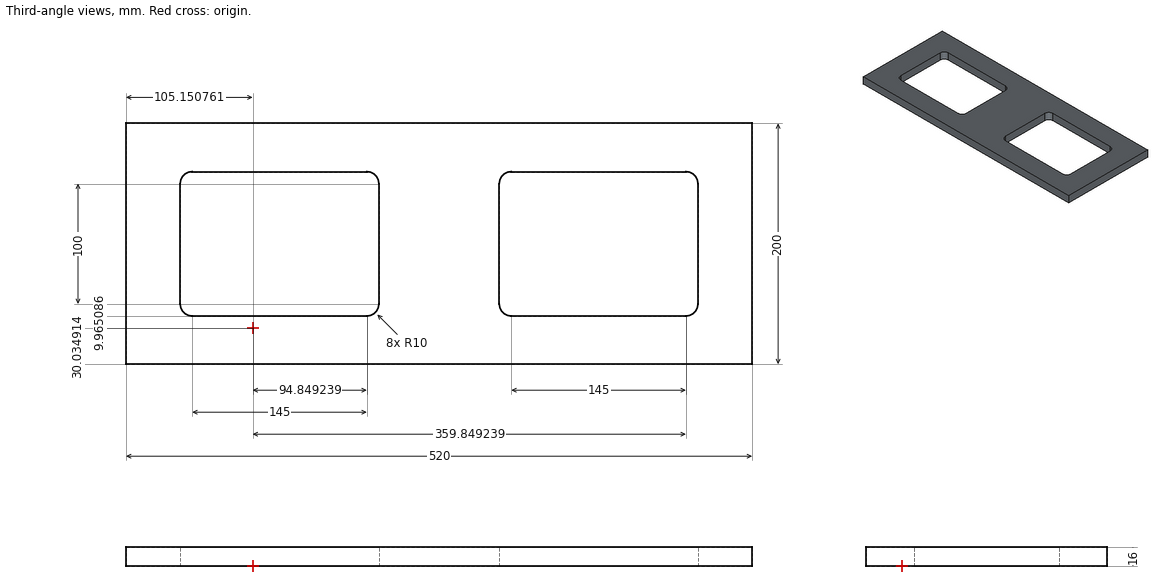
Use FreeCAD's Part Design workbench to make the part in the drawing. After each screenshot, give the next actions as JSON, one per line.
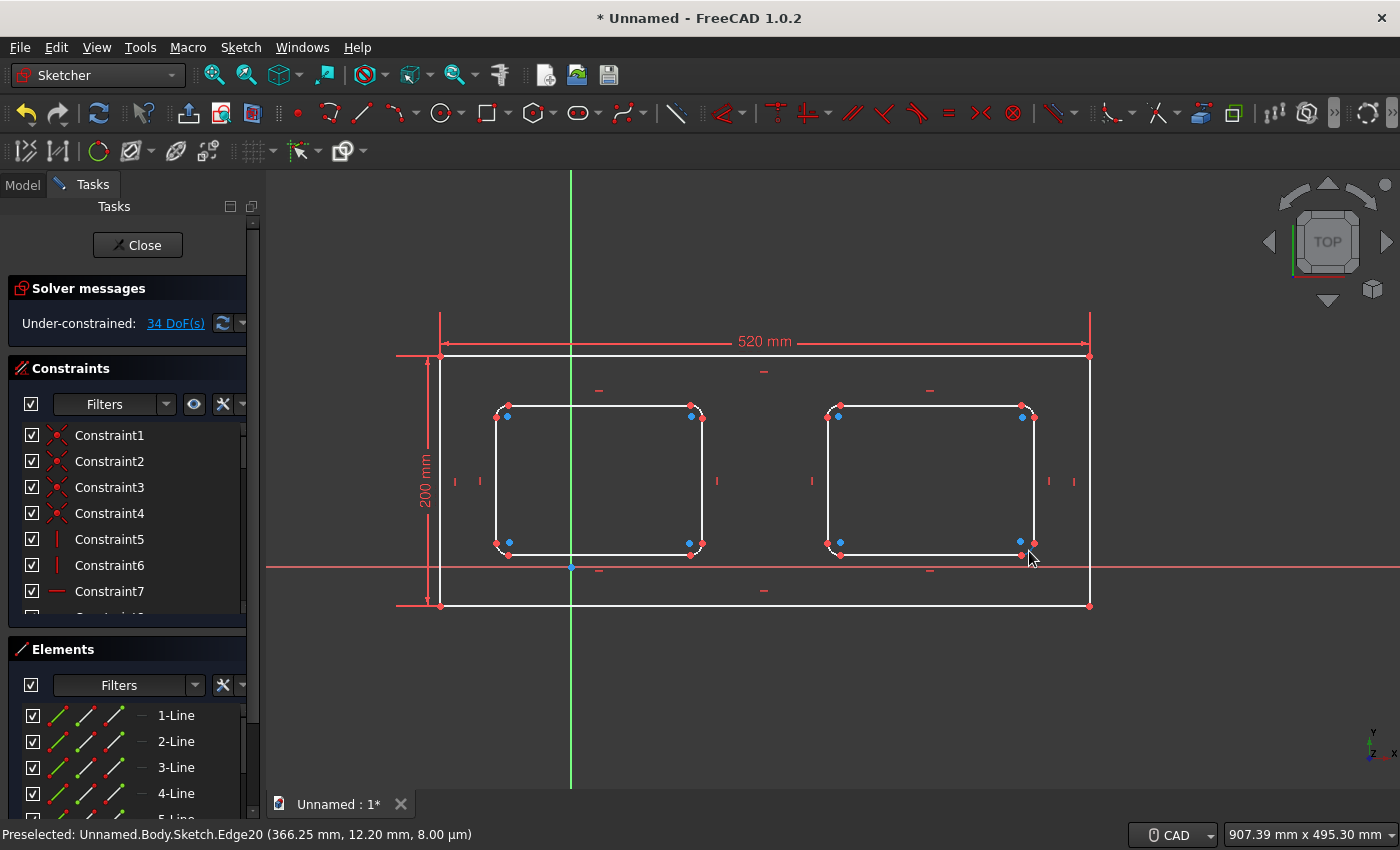
{"action": "left_click", "coordinate": [702, 456]}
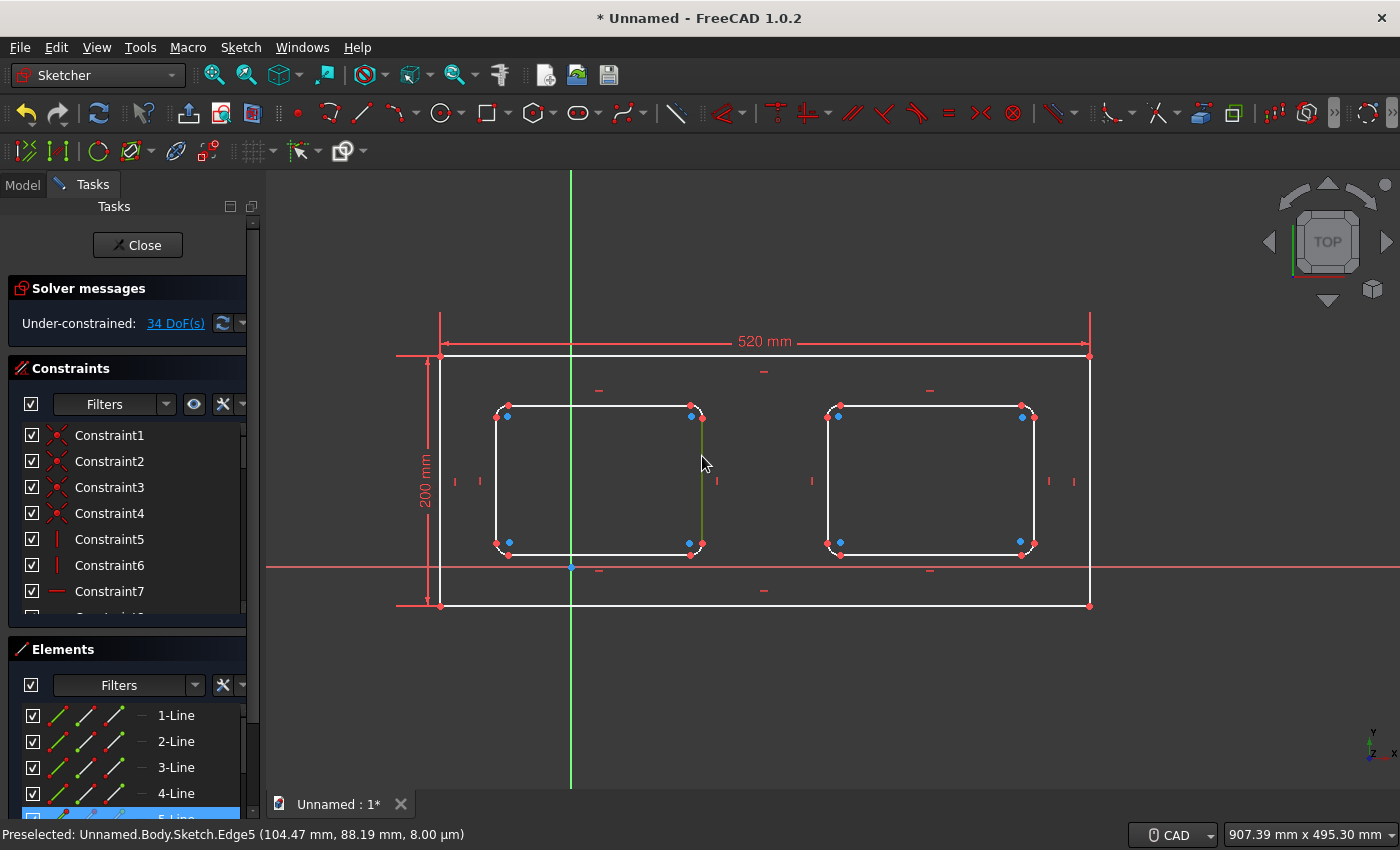
{"action": "scroll", "coordinate": [699, 552], "scroll_direction": "up", "scroll_amount": 3}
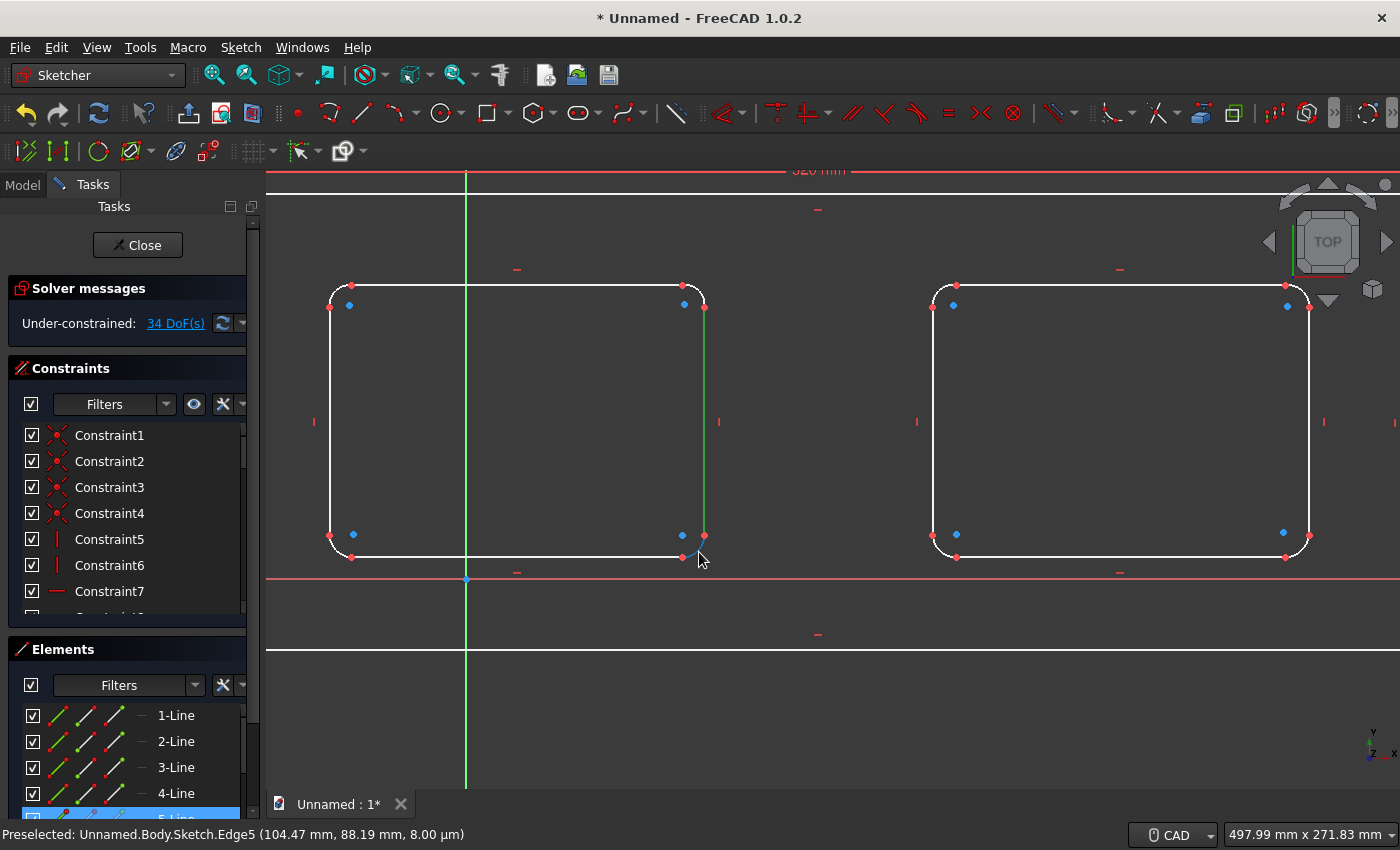
{"action": "left_click", "coordinate": [698, 551]}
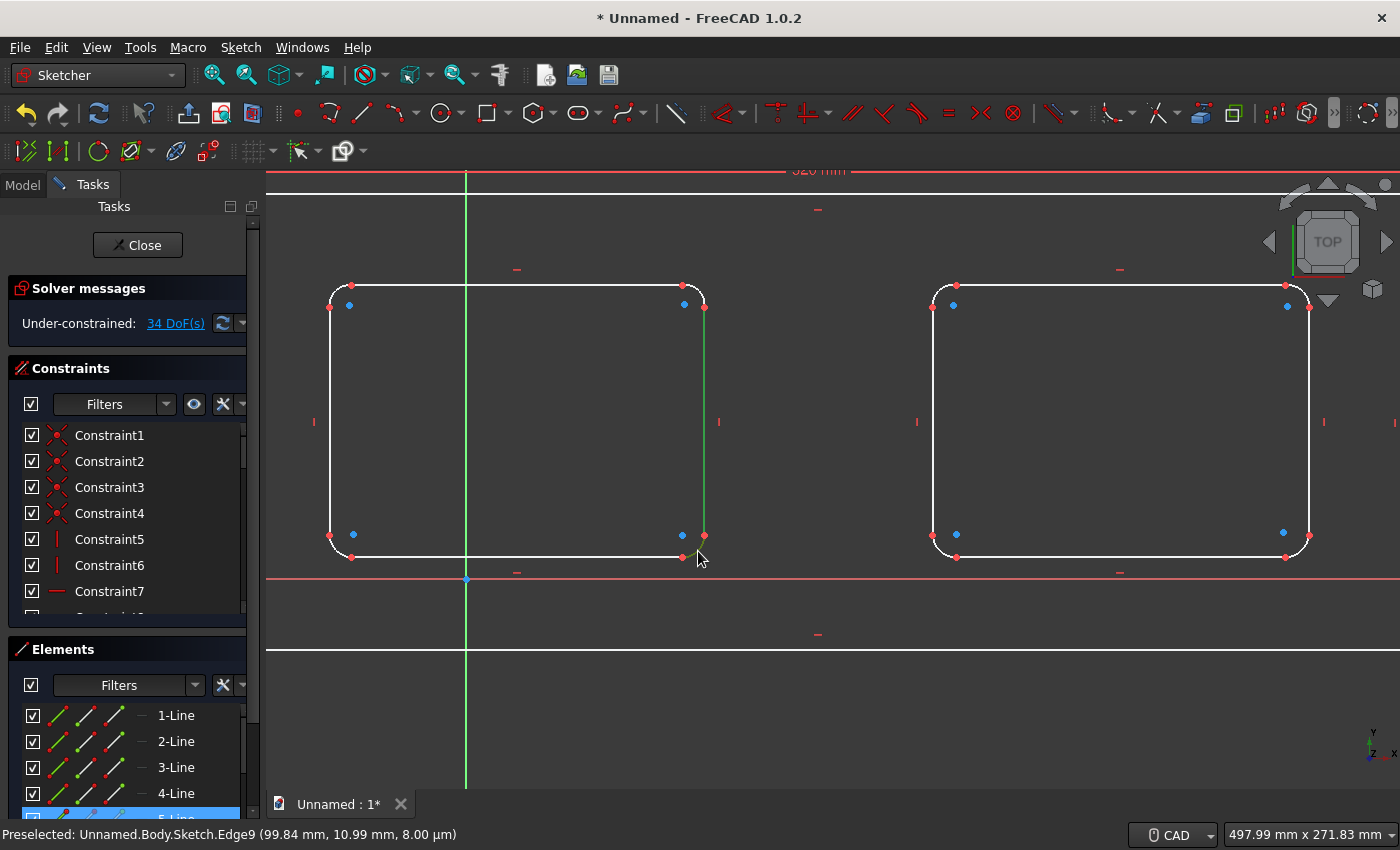
{"action": "left_click", "coordinate": [918, 114]}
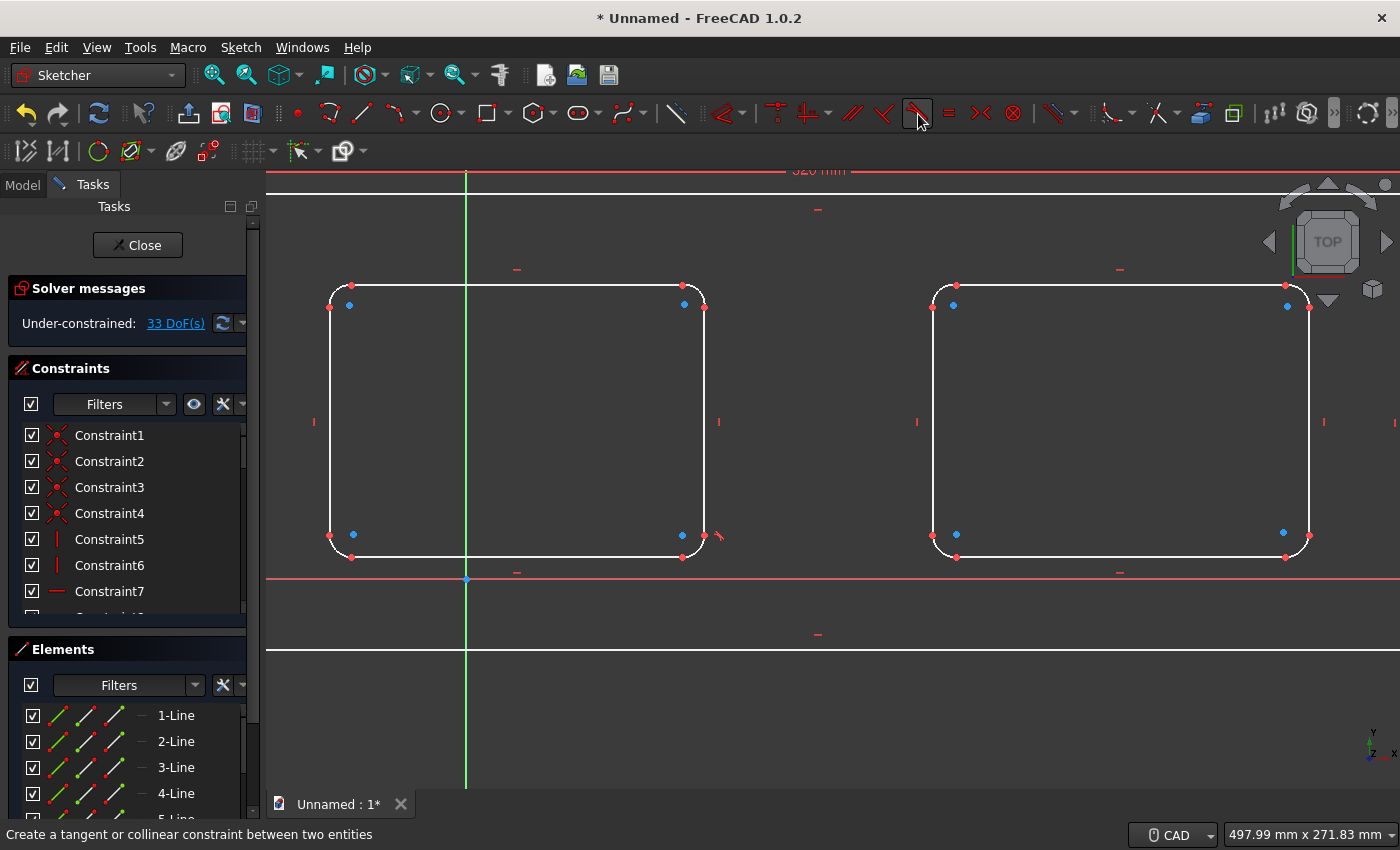
{"action": "left_click", "coordinate": [704, 376]}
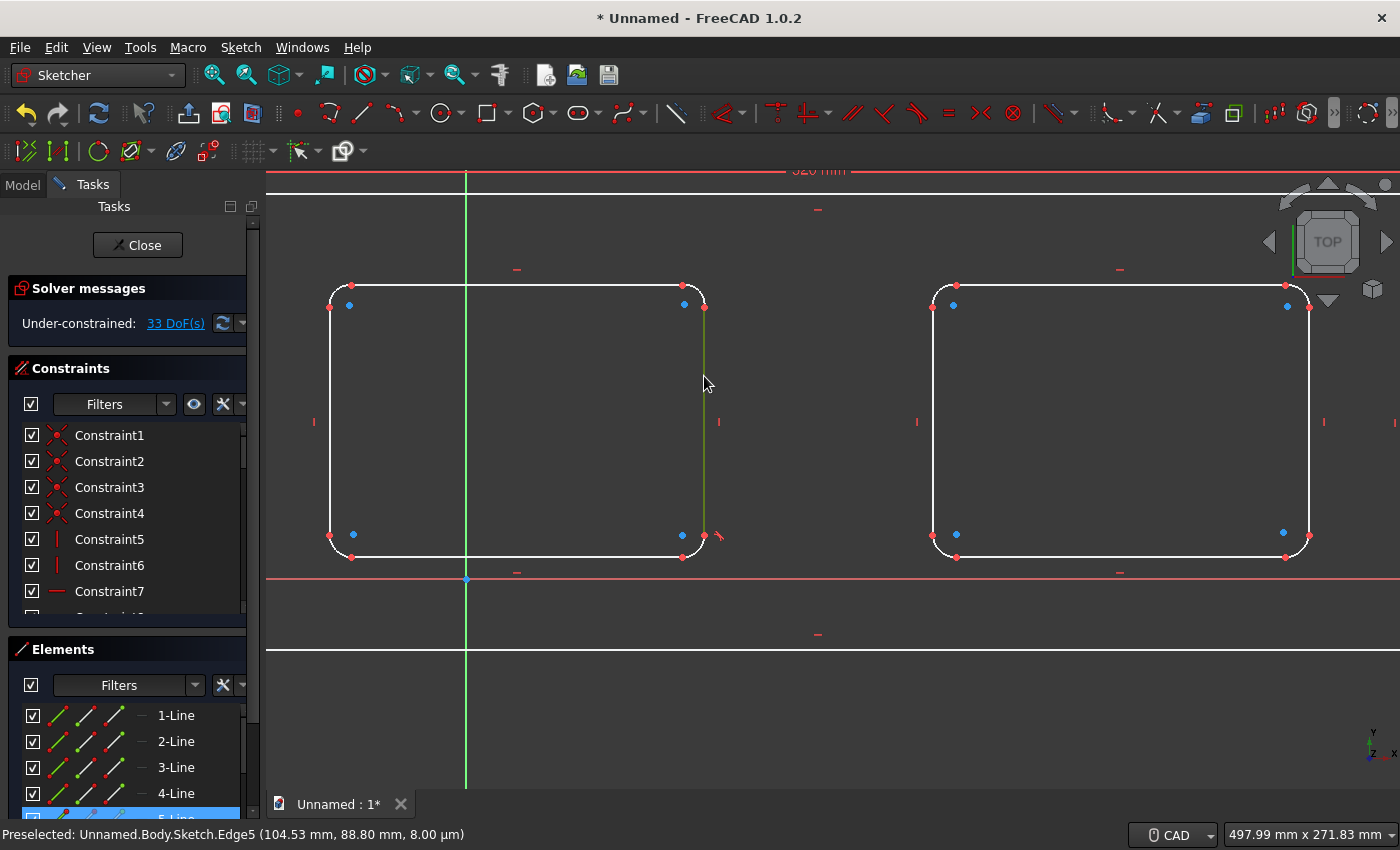
{"action": "scroll", "coordinate": [703, 297], "scroll_direction": "up", "scroll_amount": 2}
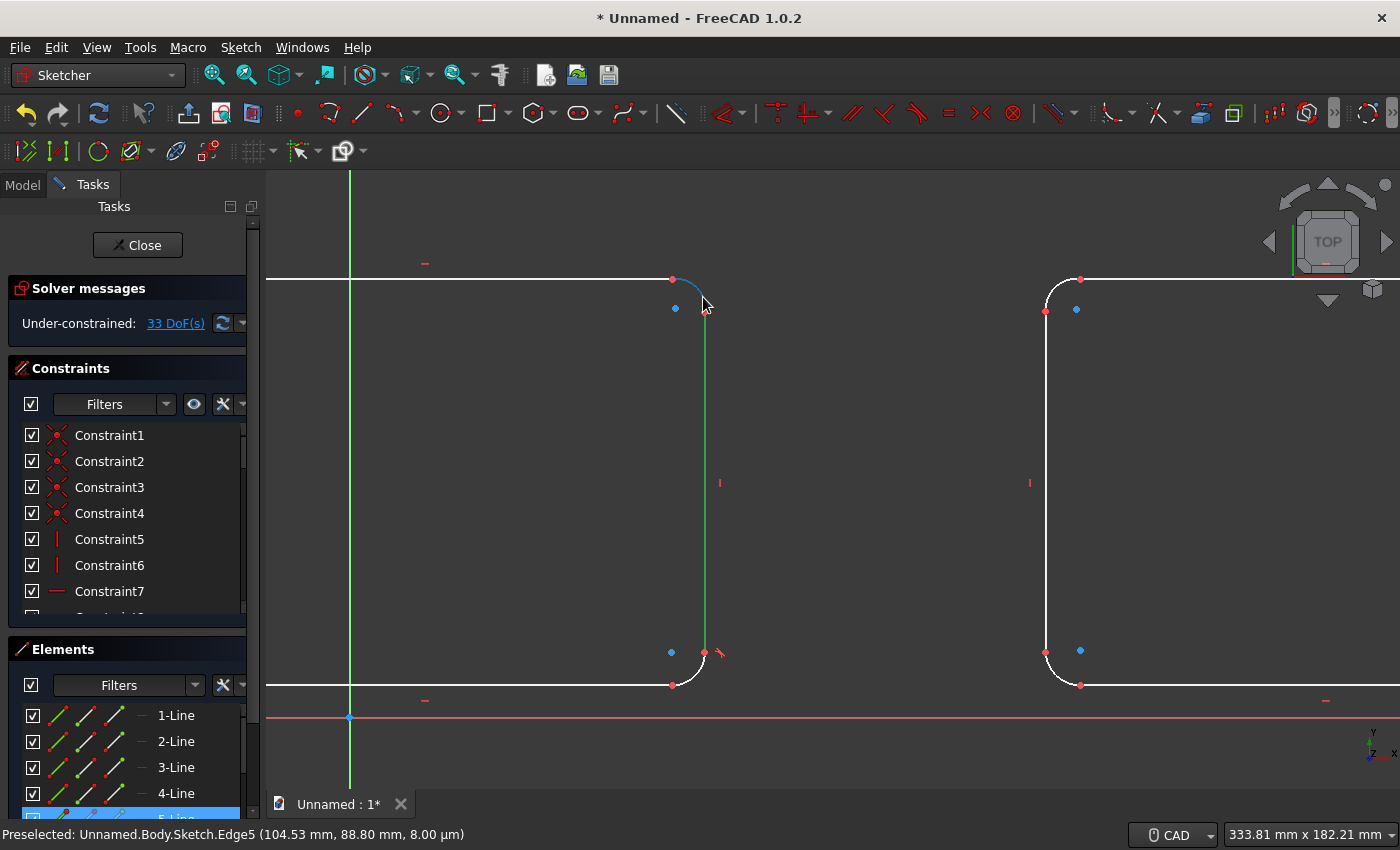
{"action": "left_click", "coordinate": [703, 297]}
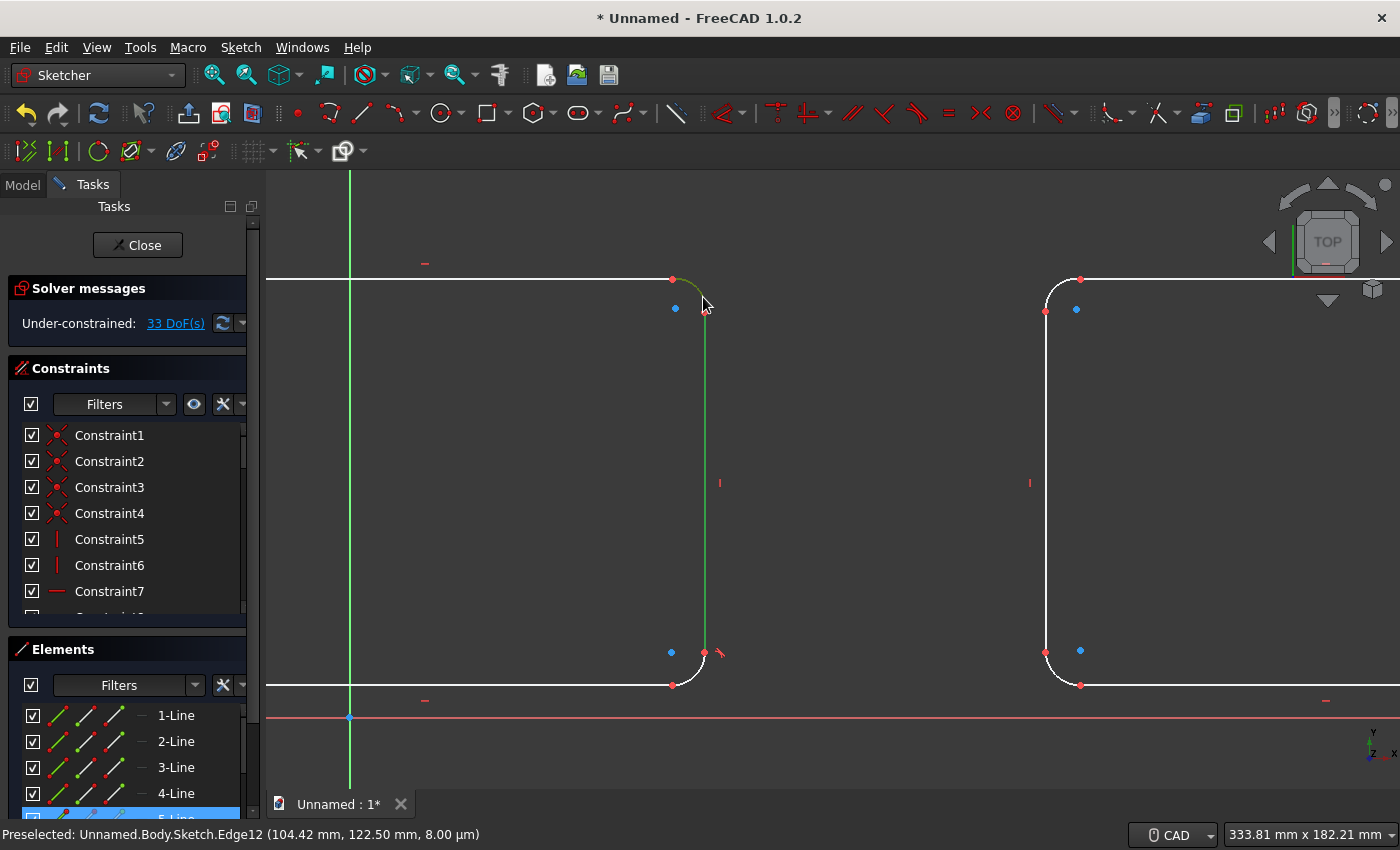
{"action": "left_click", "coordinate": [918, 114]}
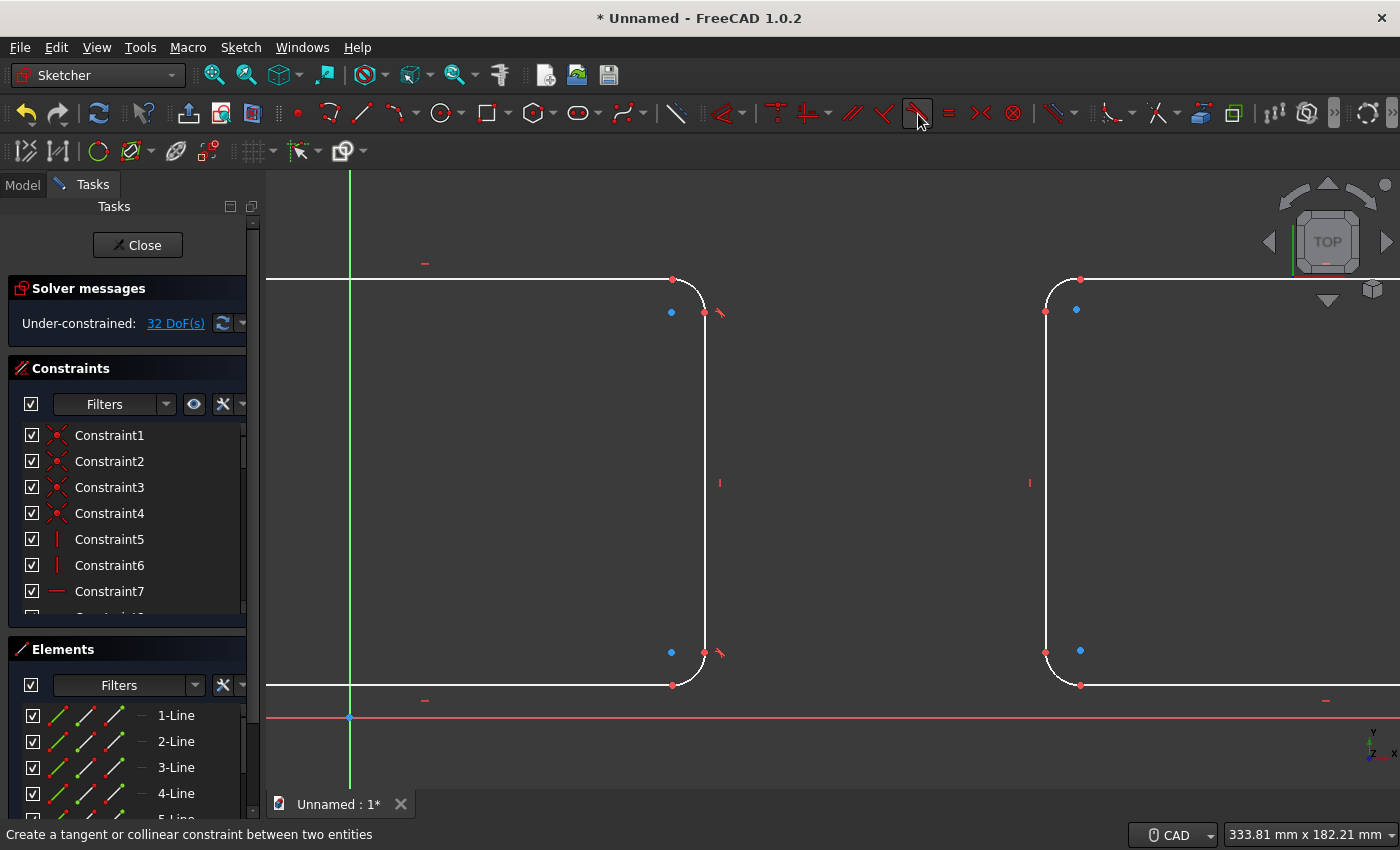
{"action": "left_click", "coordinate": [524, 685]}